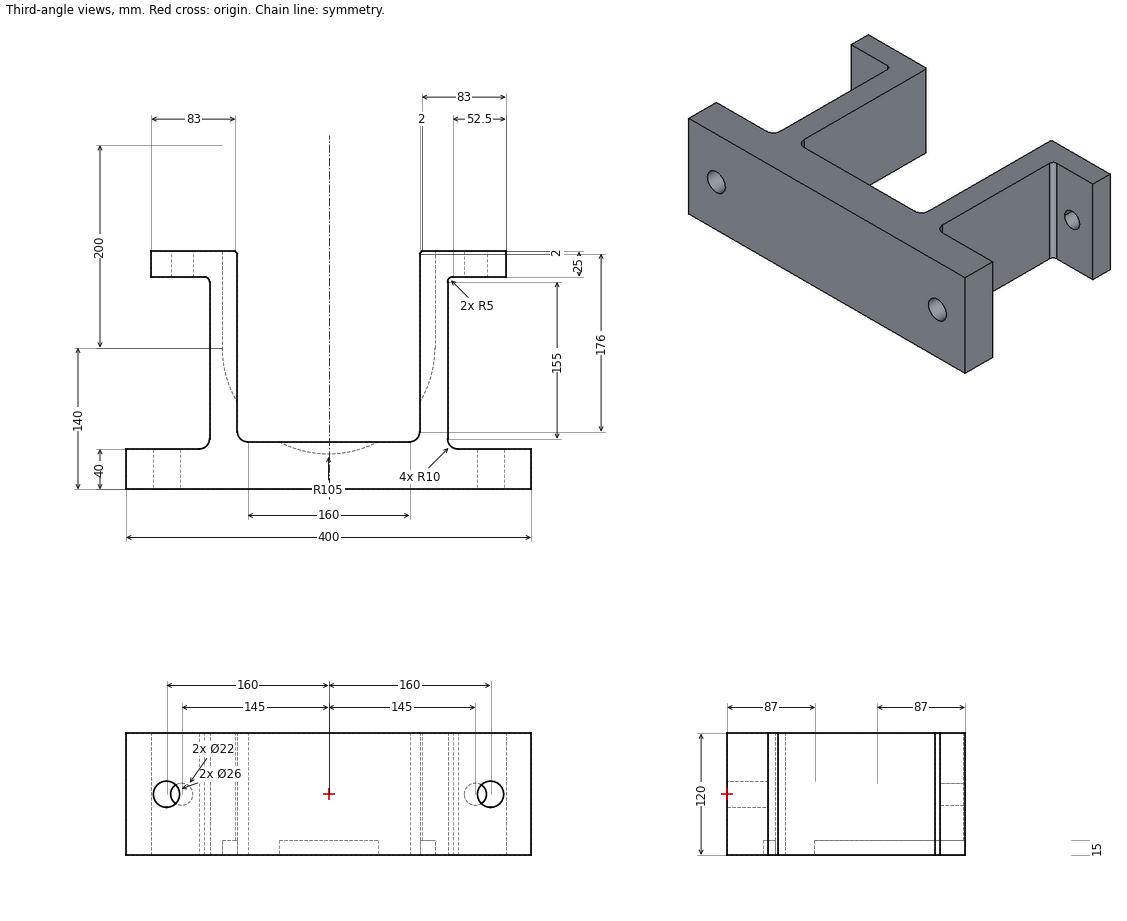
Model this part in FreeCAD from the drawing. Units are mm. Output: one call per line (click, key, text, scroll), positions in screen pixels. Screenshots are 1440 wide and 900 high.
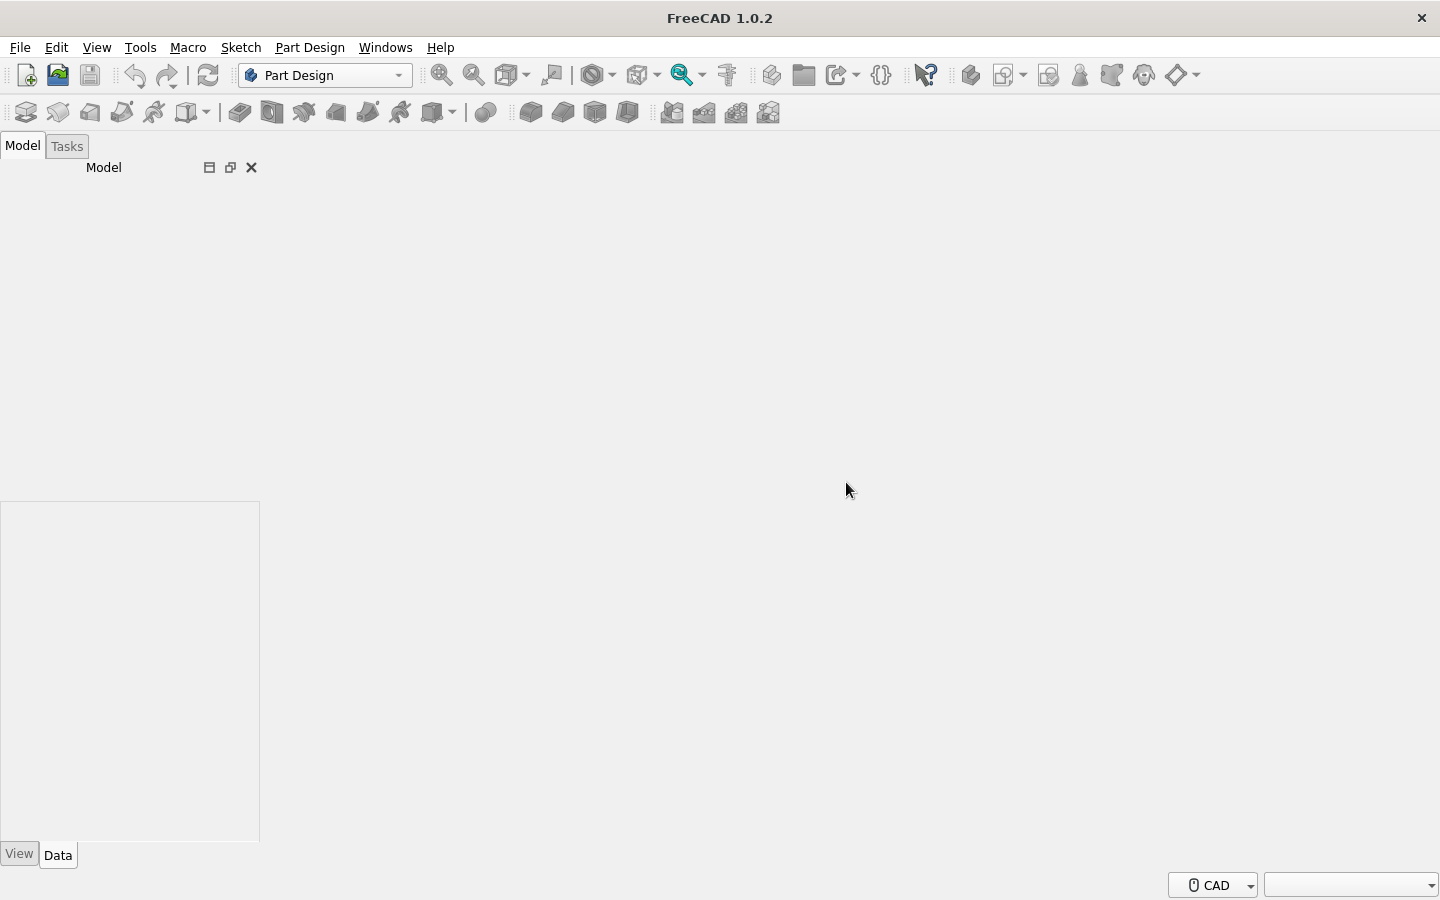
click(26, 76)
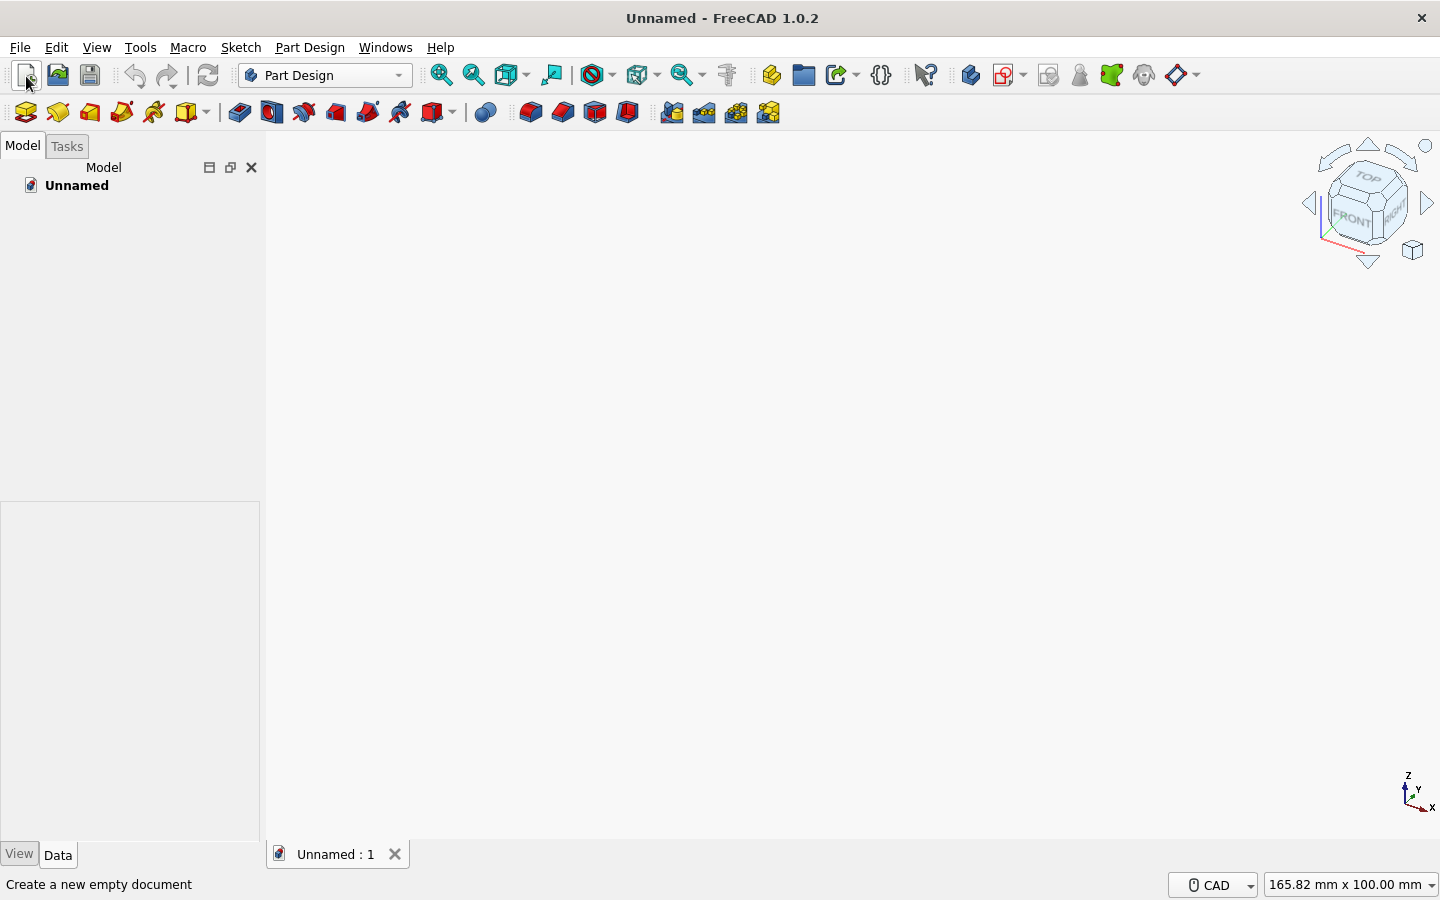
click(1004, 76)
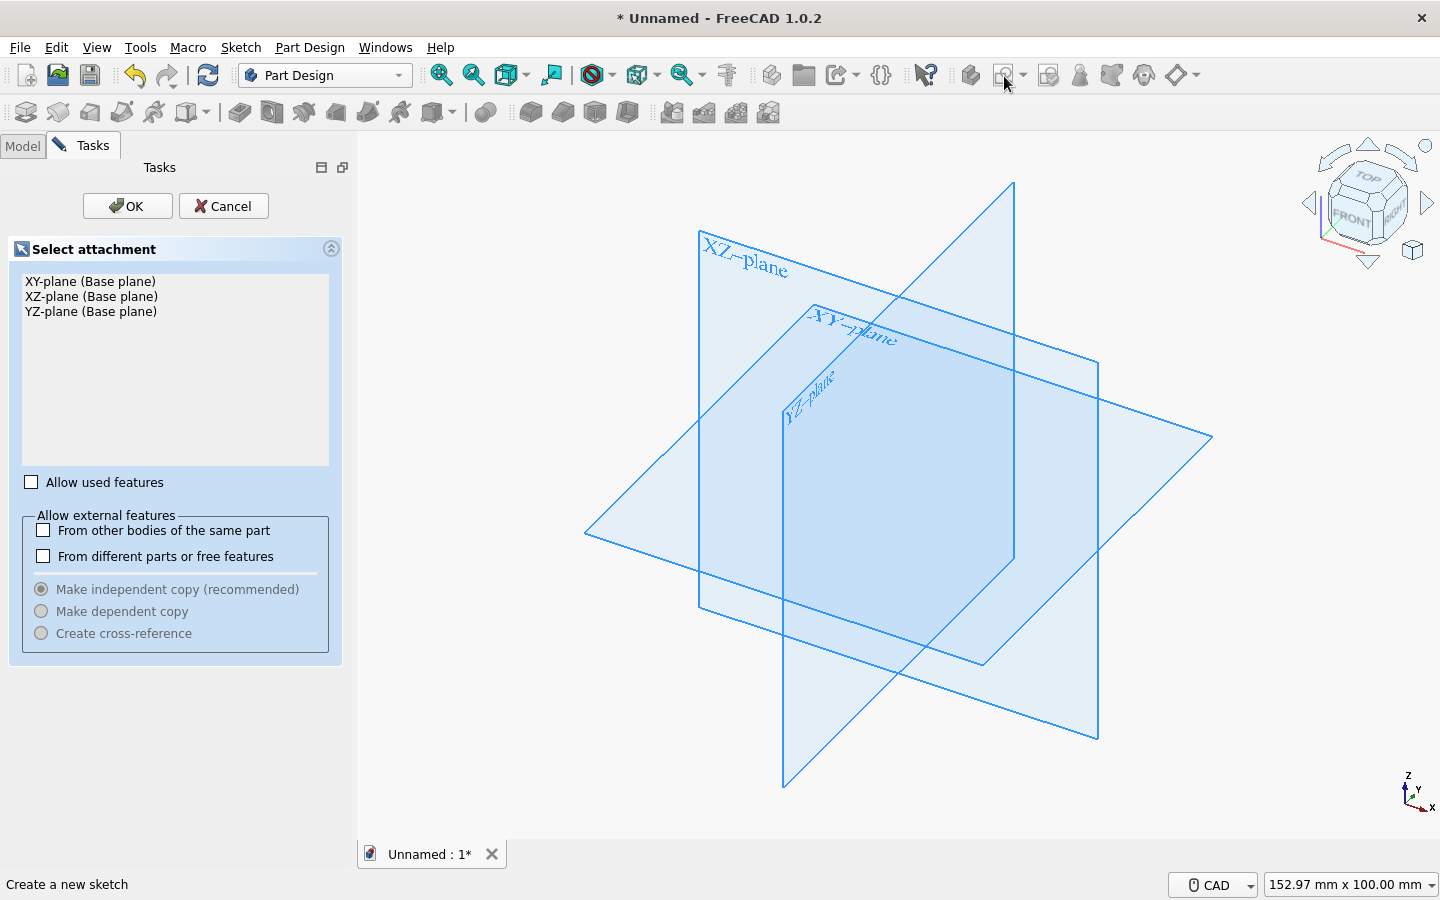
click(82, 282)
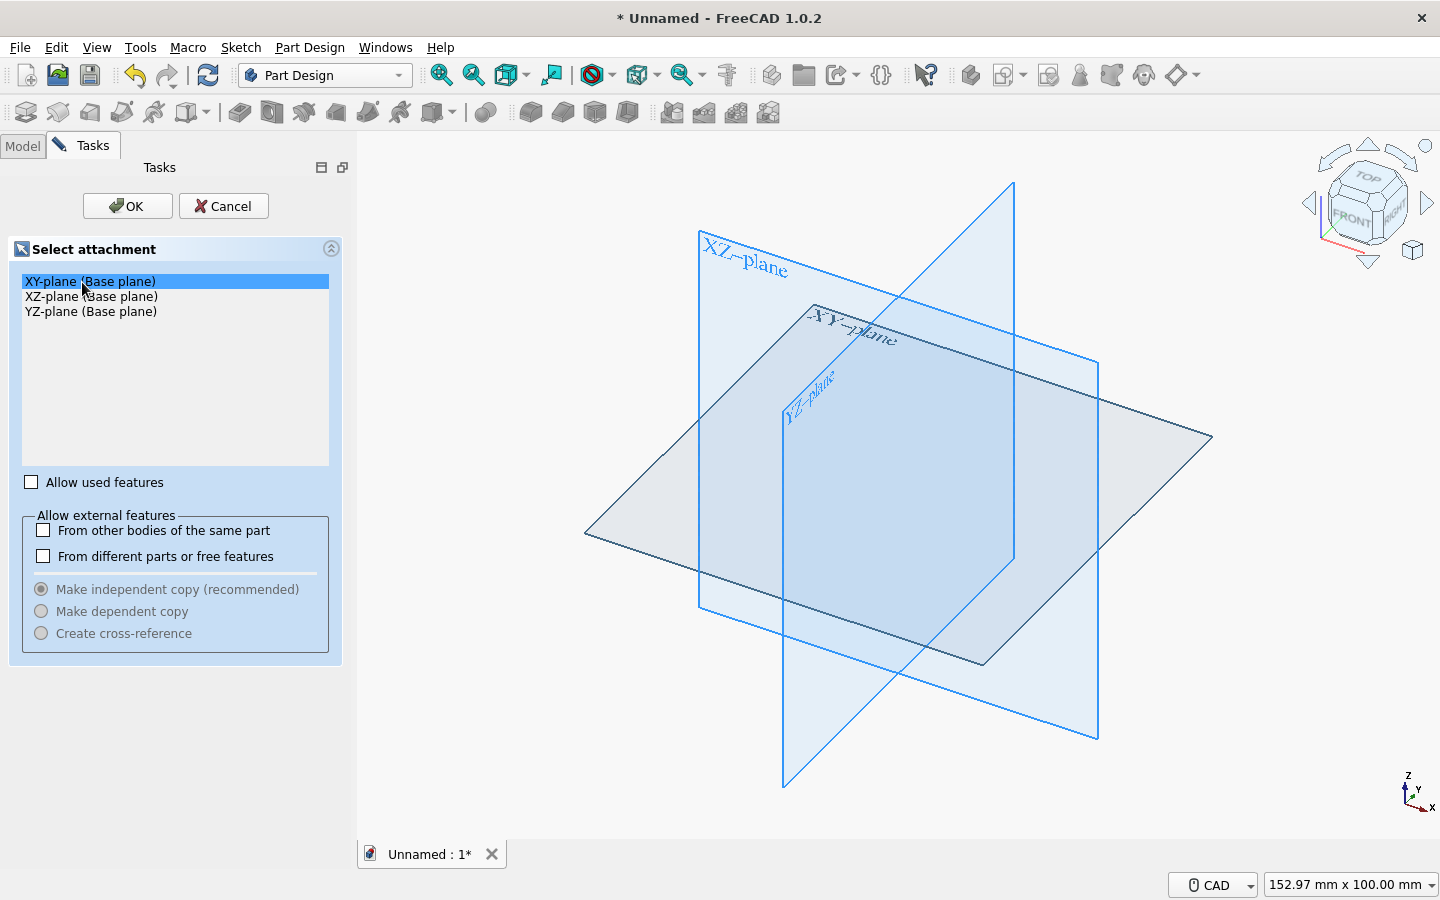
click(128, 206)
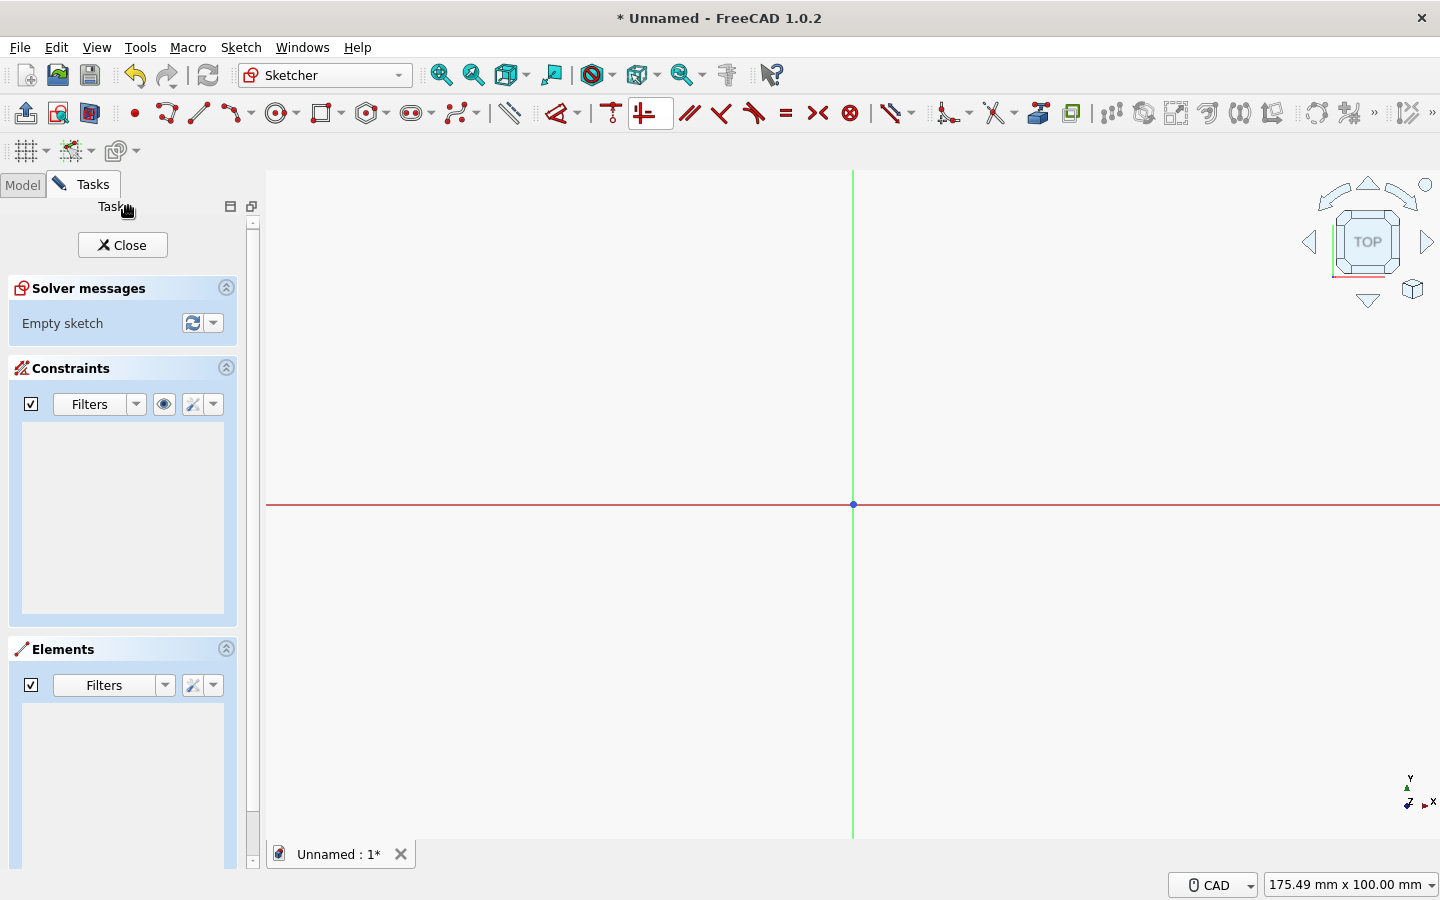
scroll(762, 762, down, 7)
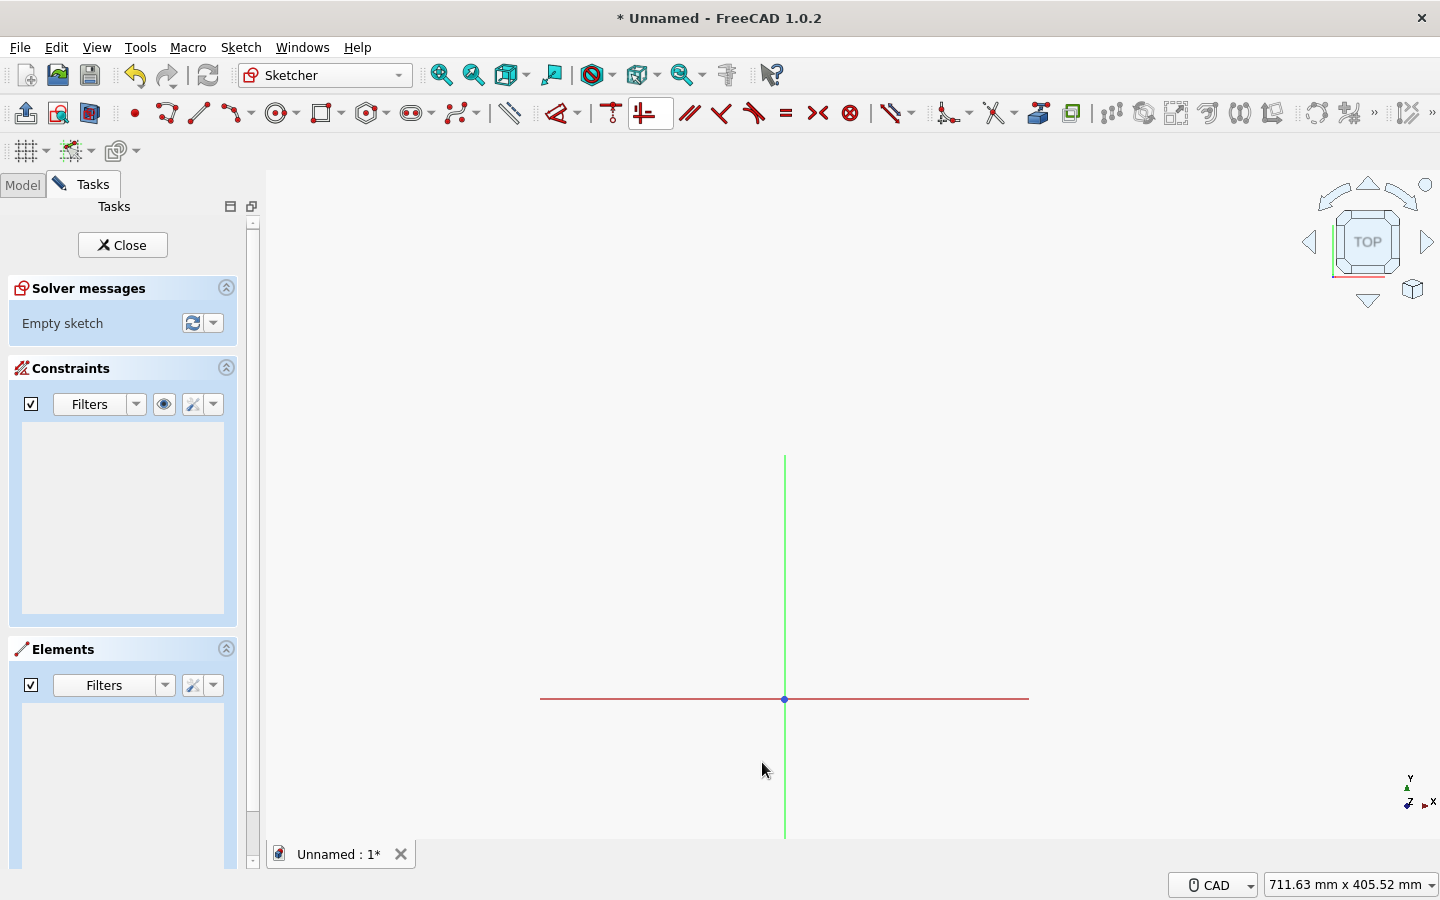
click(200, 114)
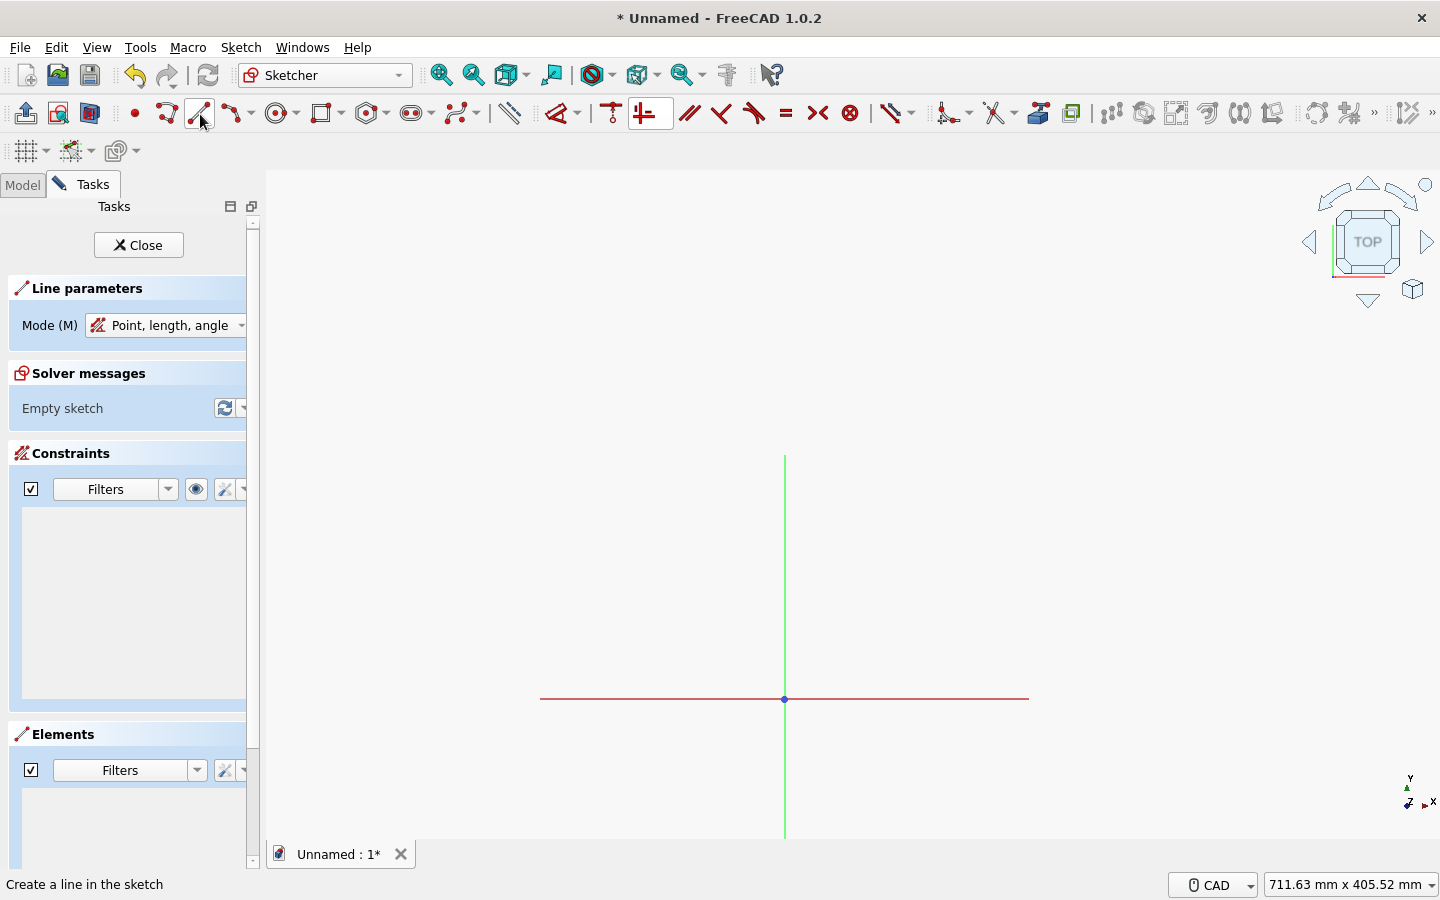
click(979, 617)
click(979, 361)